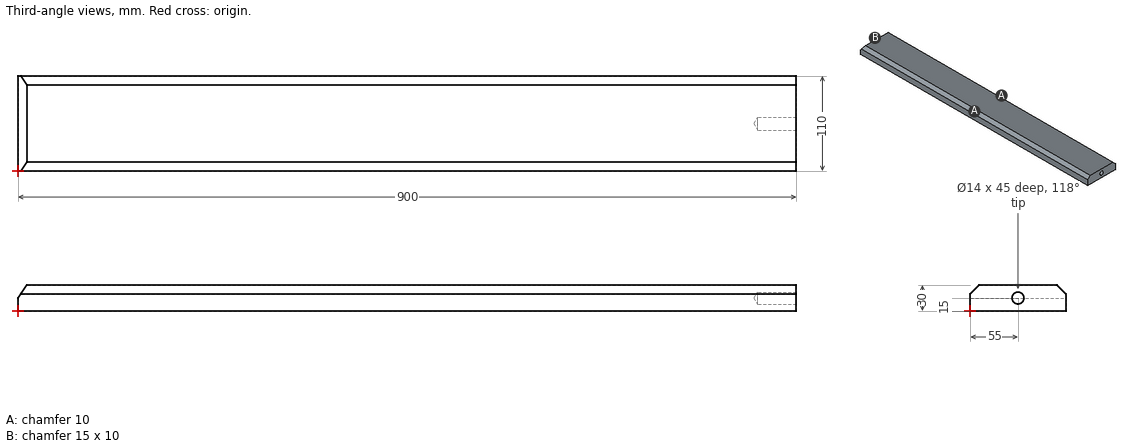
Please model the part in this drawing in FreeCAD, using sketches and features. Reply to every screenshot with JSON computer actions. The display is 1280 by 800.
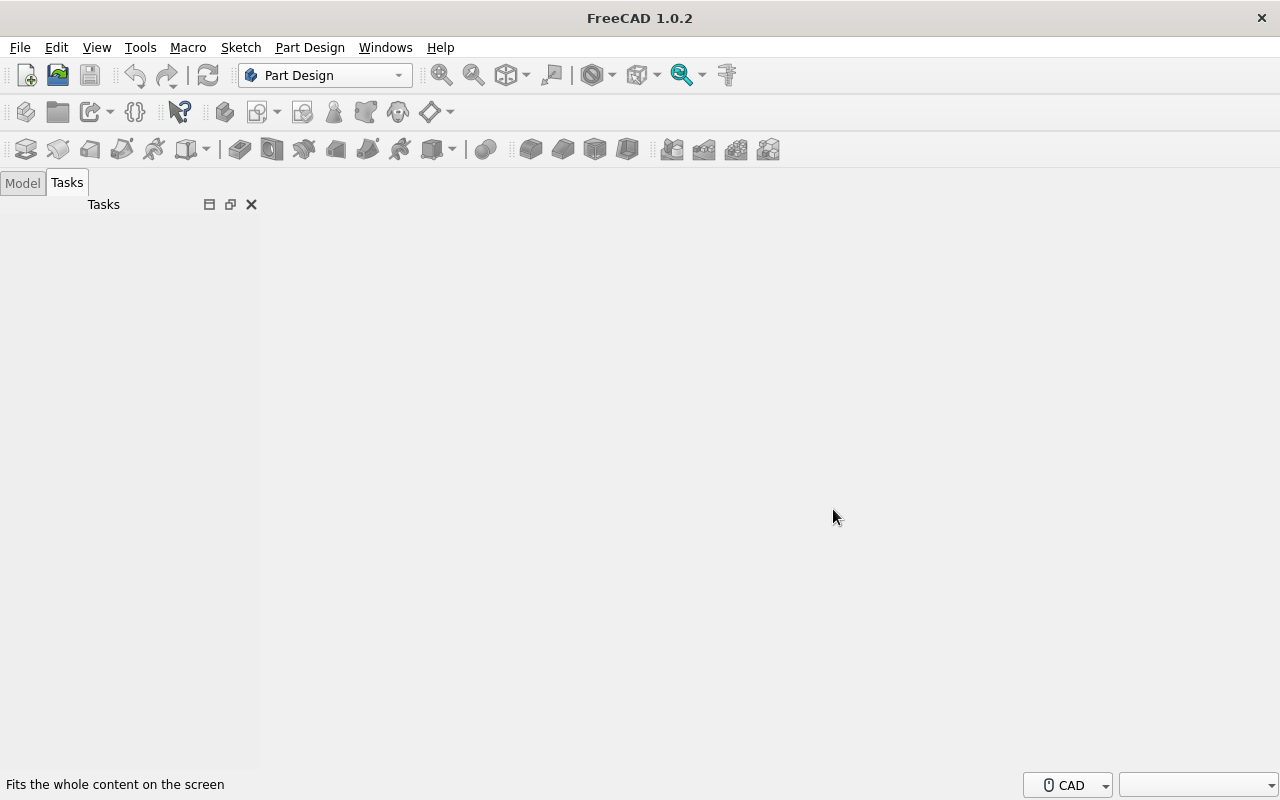
{"action": "key", "text": "ctrl+n"}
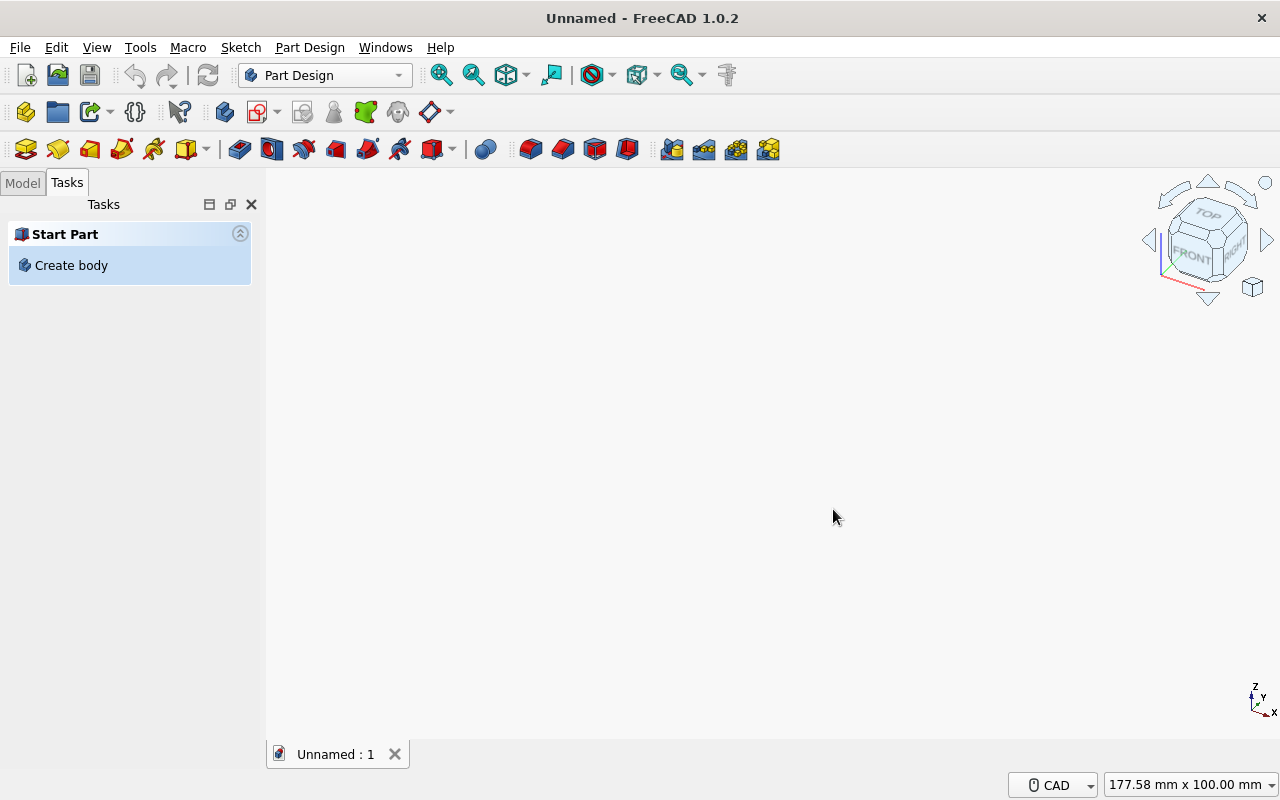
{"action": "left_click", "coordinate": [258, 112]}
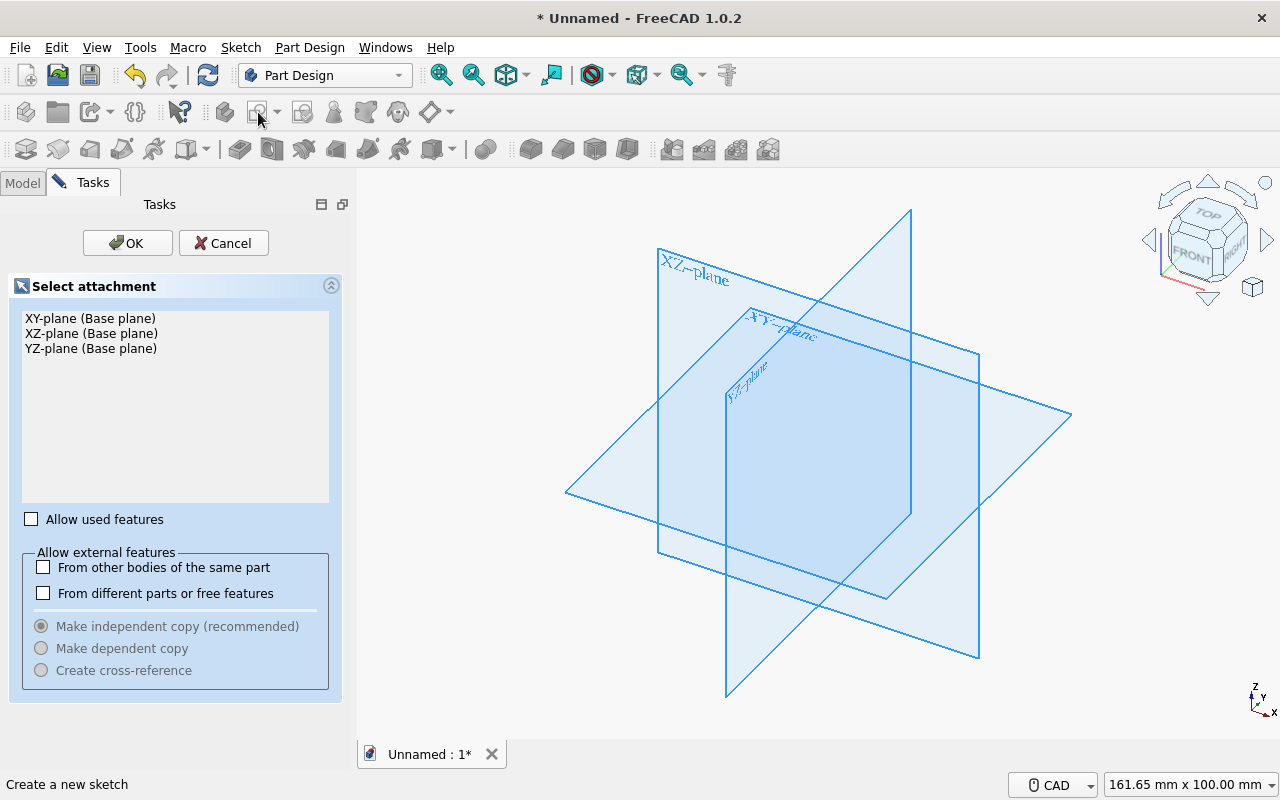
{"action": "left_click", "coordinate": [82, 318]}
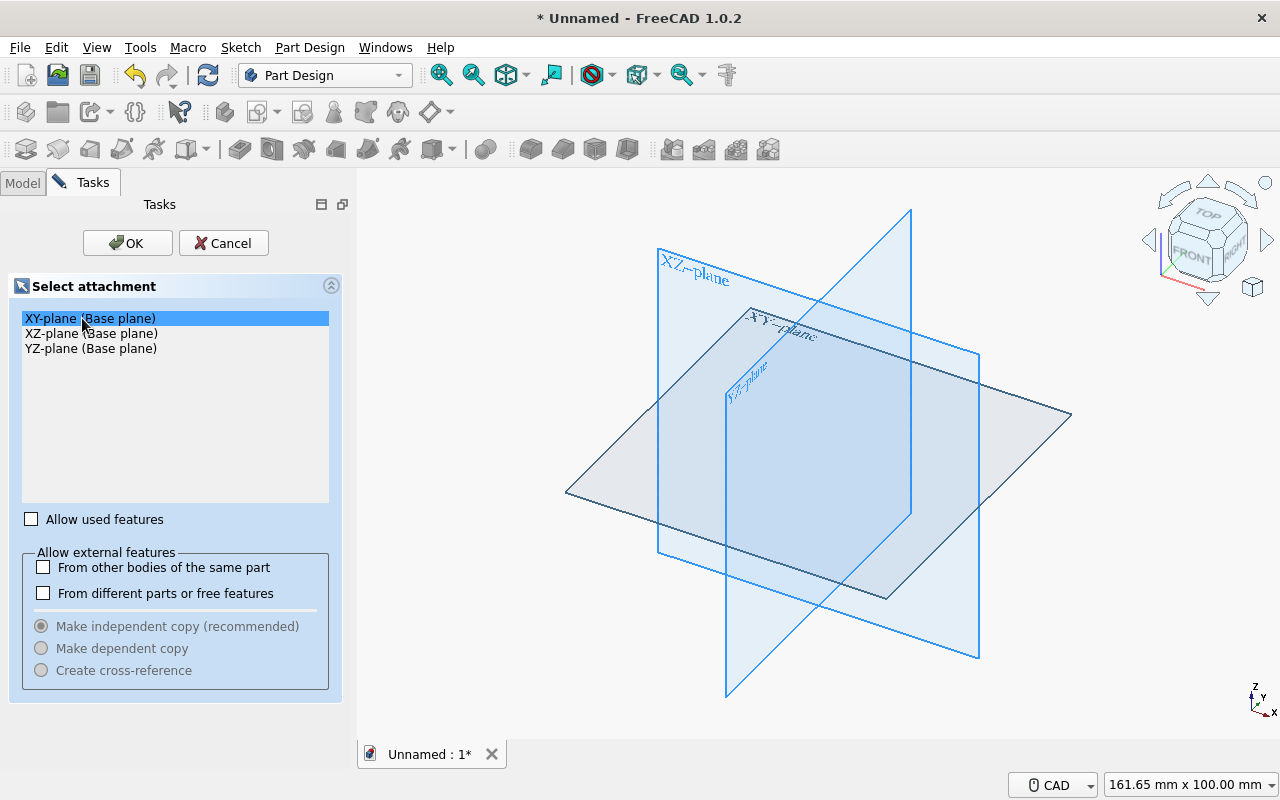
{"action": "left_click", "coordinate": [128, 243]}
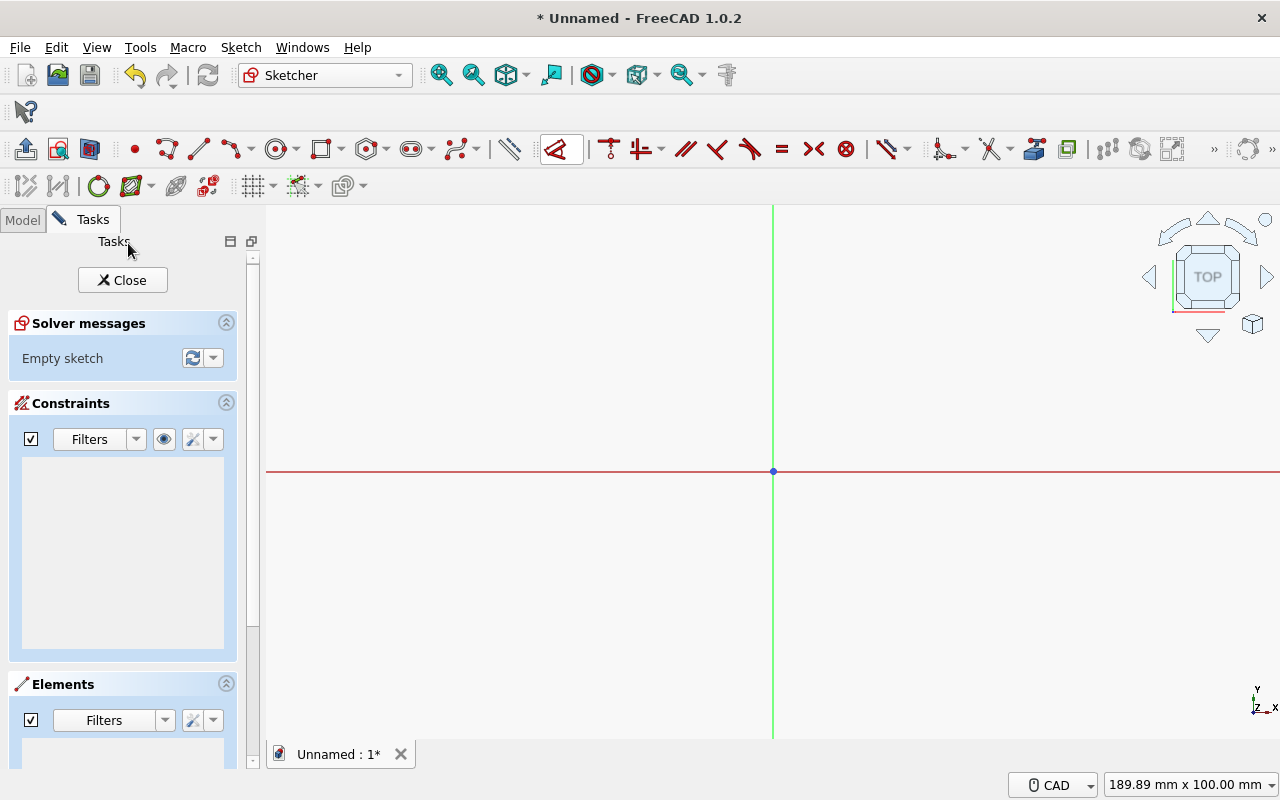
{"action": "scroll", "coordinate": [397, 509], "scroll_direction": "down", "scroll_amount": 11}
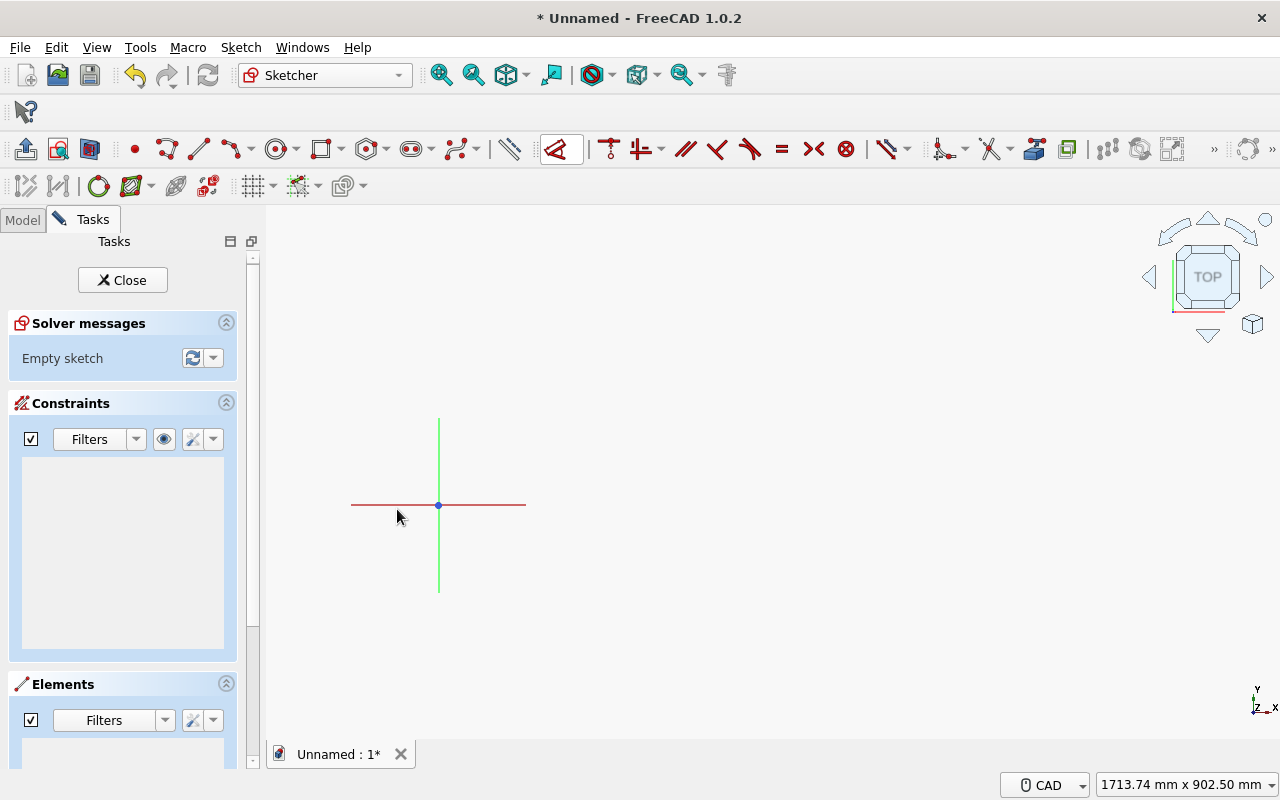
{"action": "key", "text": "g r"}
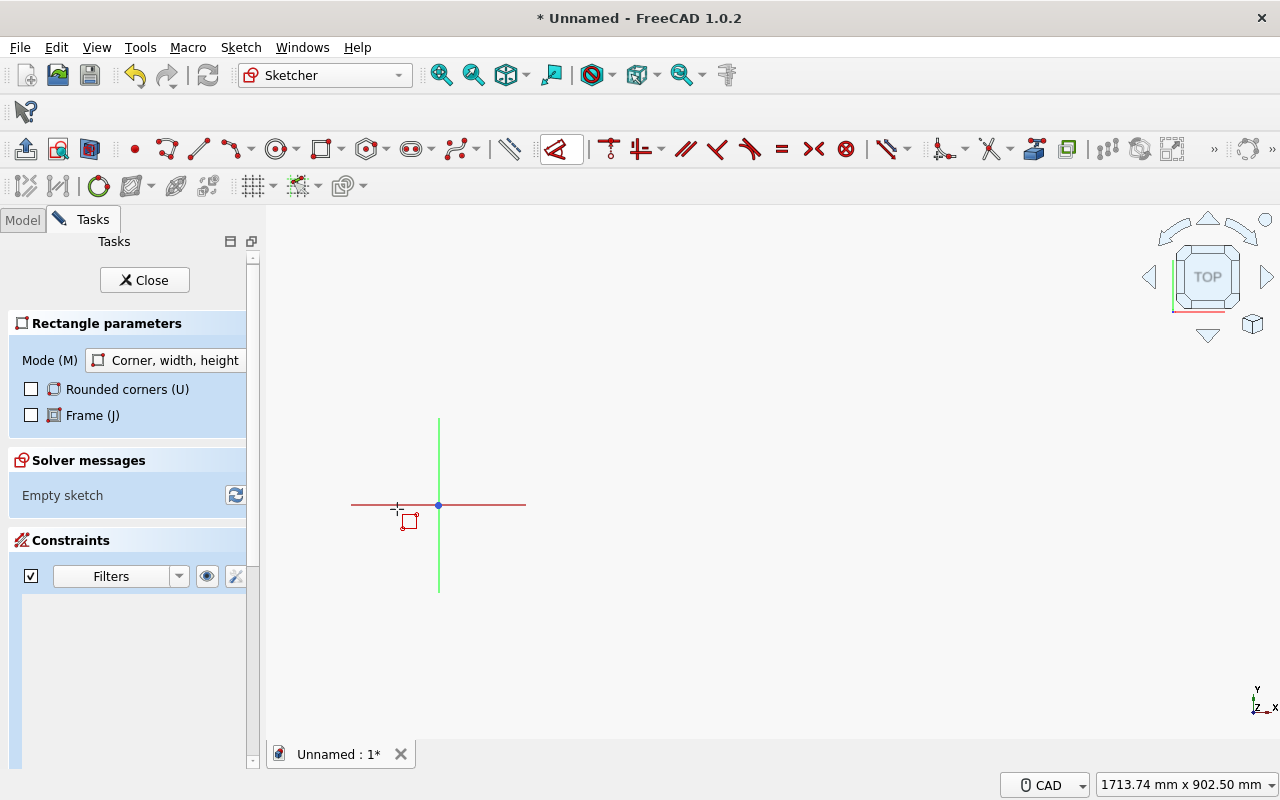
{"action": "left_click", "coordinate": [439, 505]}
{"action": "mouse_move", "coordinate": [971, 440]}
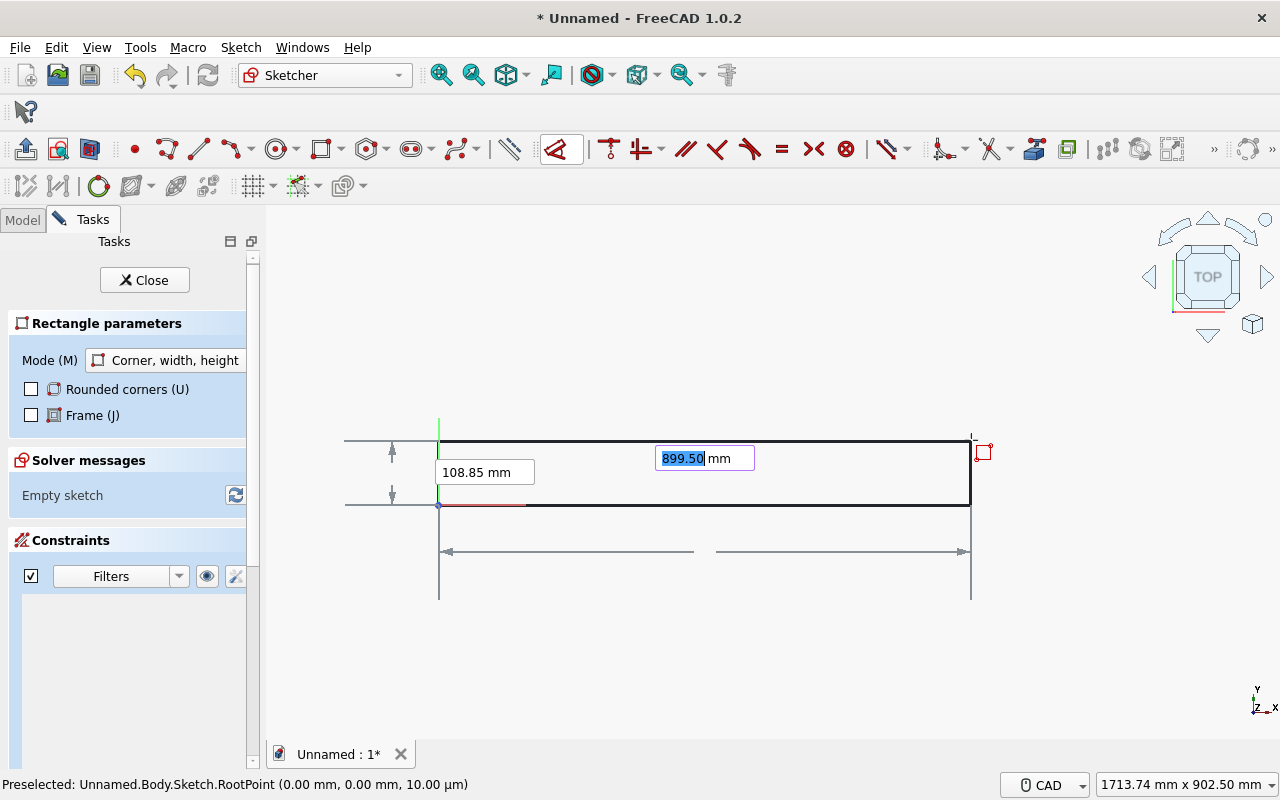
{"action": "type", "text": "900"}
{"action": "key", "text": "Tab"}
{"action": "type", "text": "110"}
{"action": "key", "text": "Return"}
{"action": "key", "text": "Escape"}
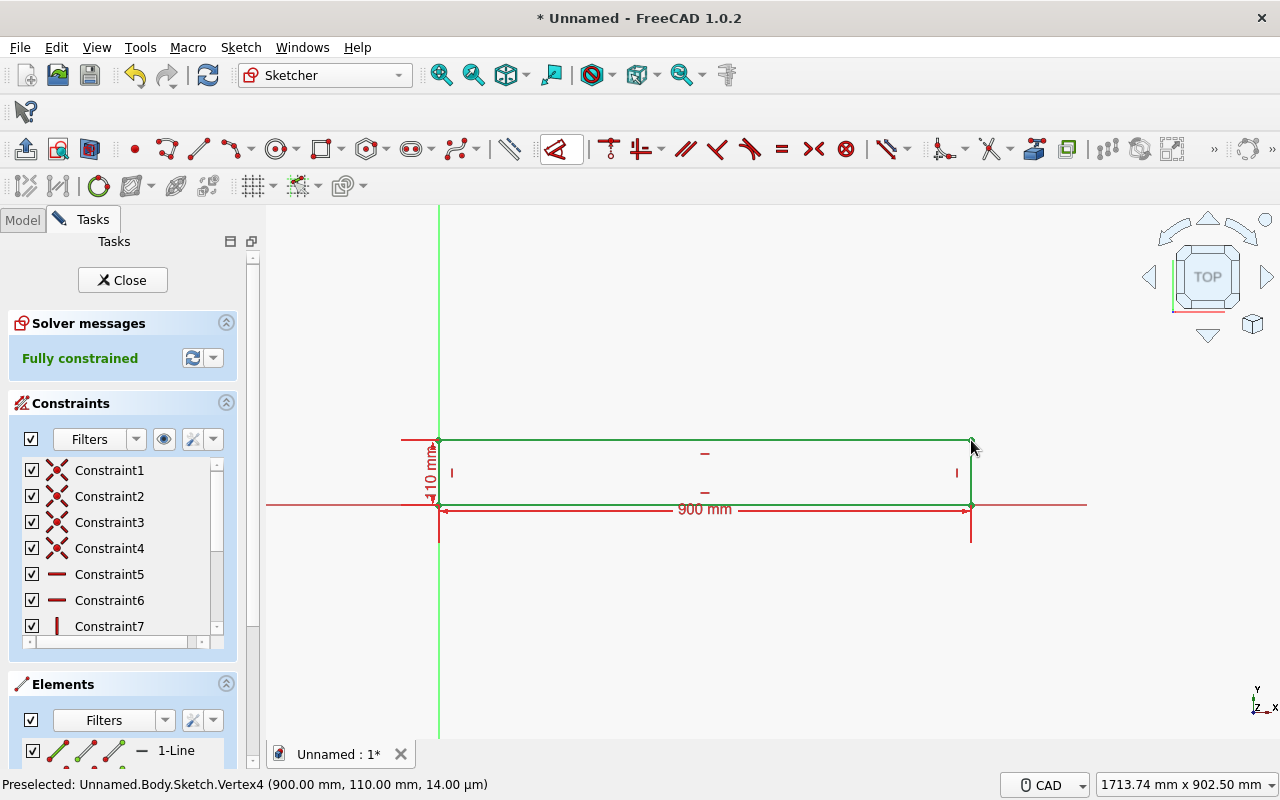
{"action": "left_click", "coordinate": [123, 280]}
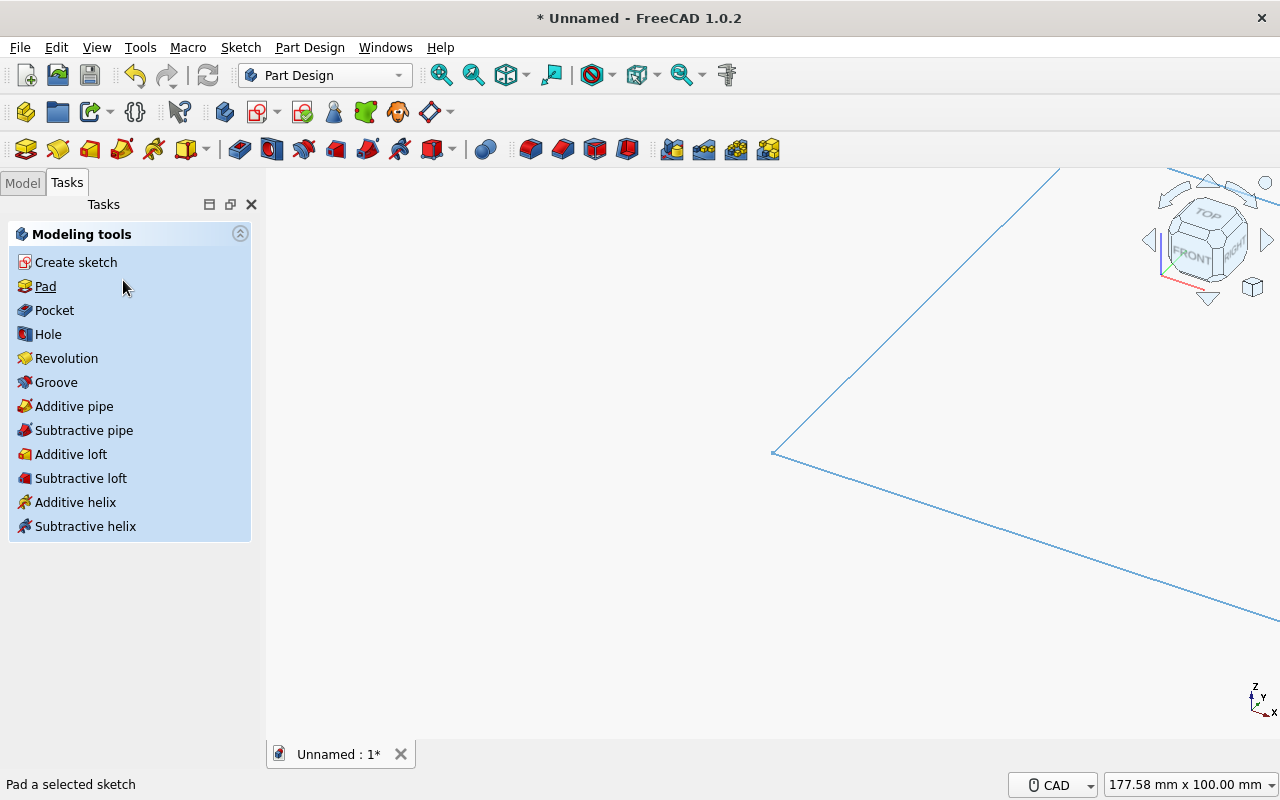
{"action": "left_click", "coordinate": [26, 150]}